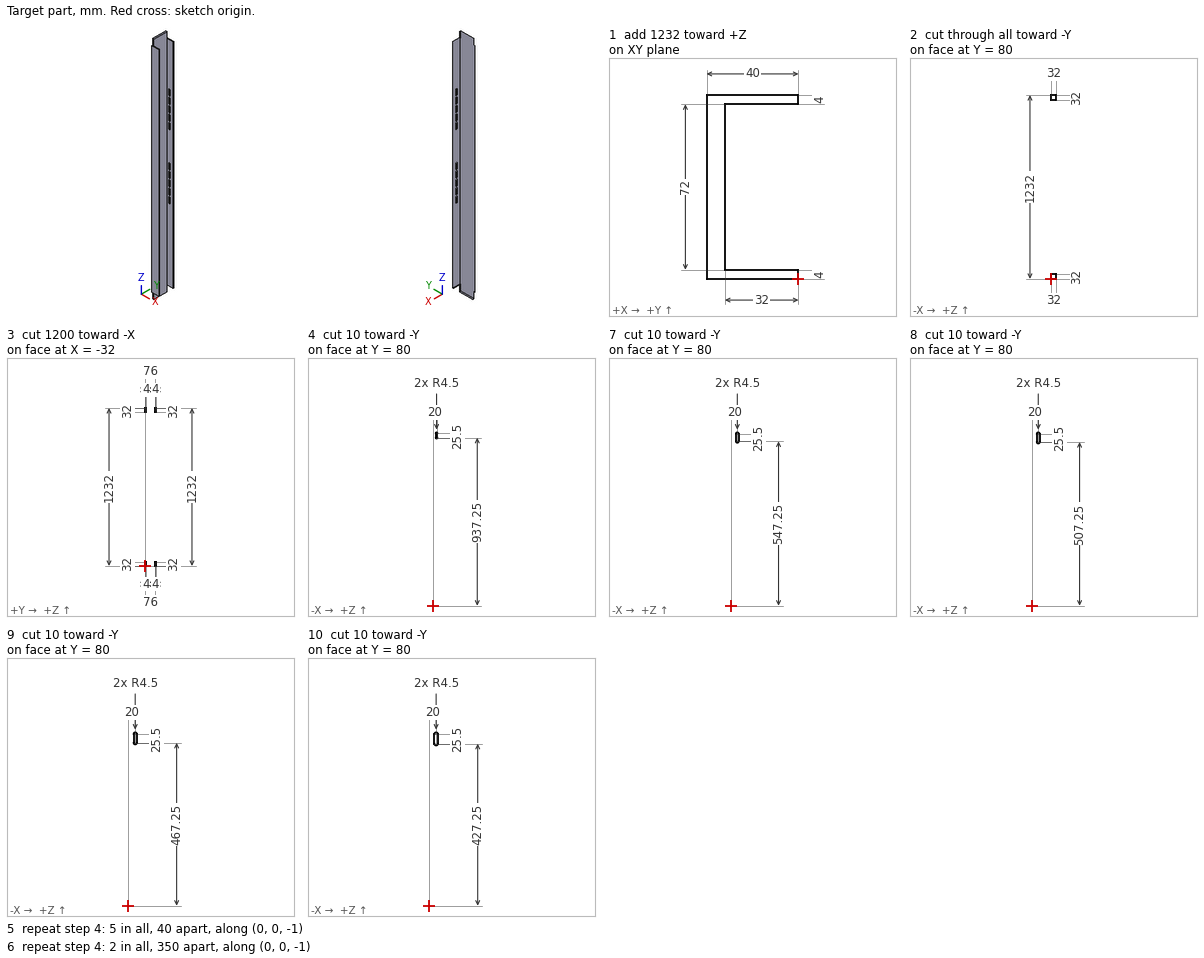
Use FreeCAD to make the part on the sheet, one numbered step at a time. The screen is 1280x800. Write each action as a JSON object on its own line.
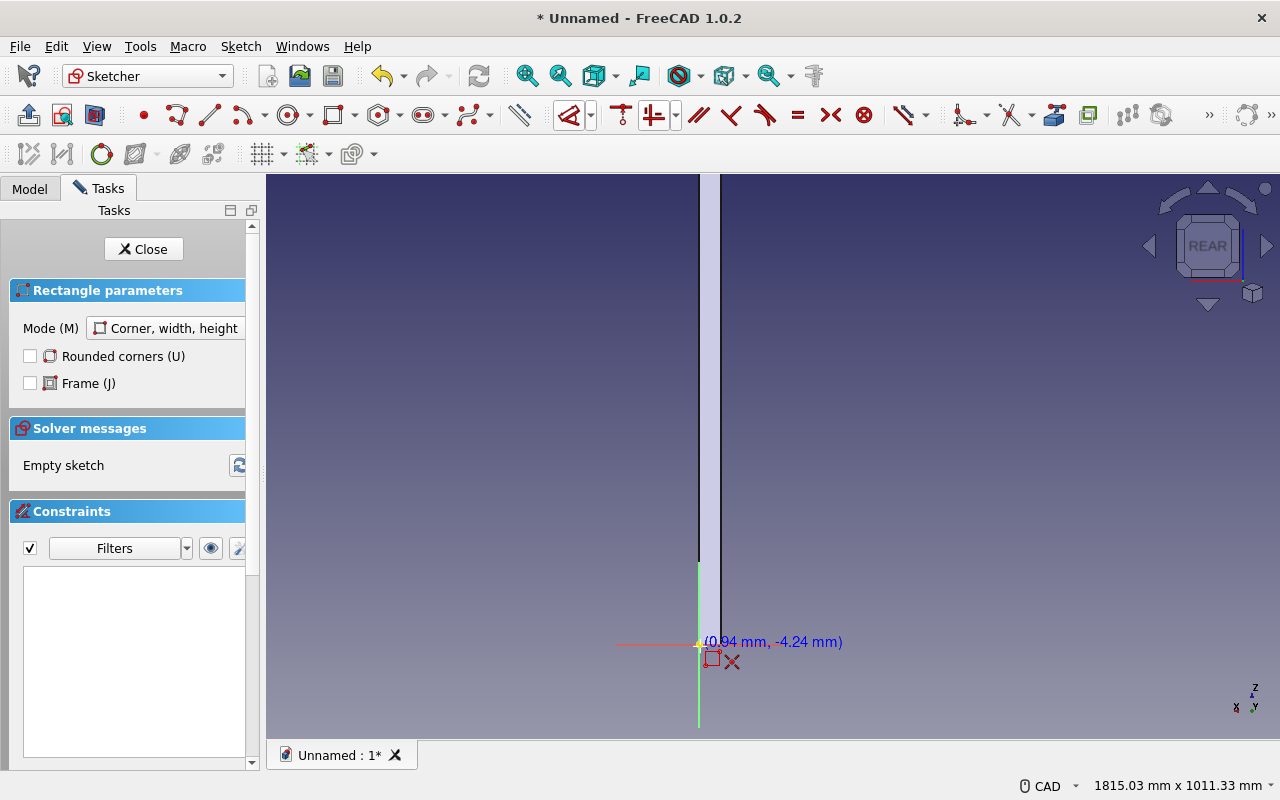
{"action": "left_click", "coordinate": [699, 645]}
{"action": "mouse_move", "coordinate": [717, 627]}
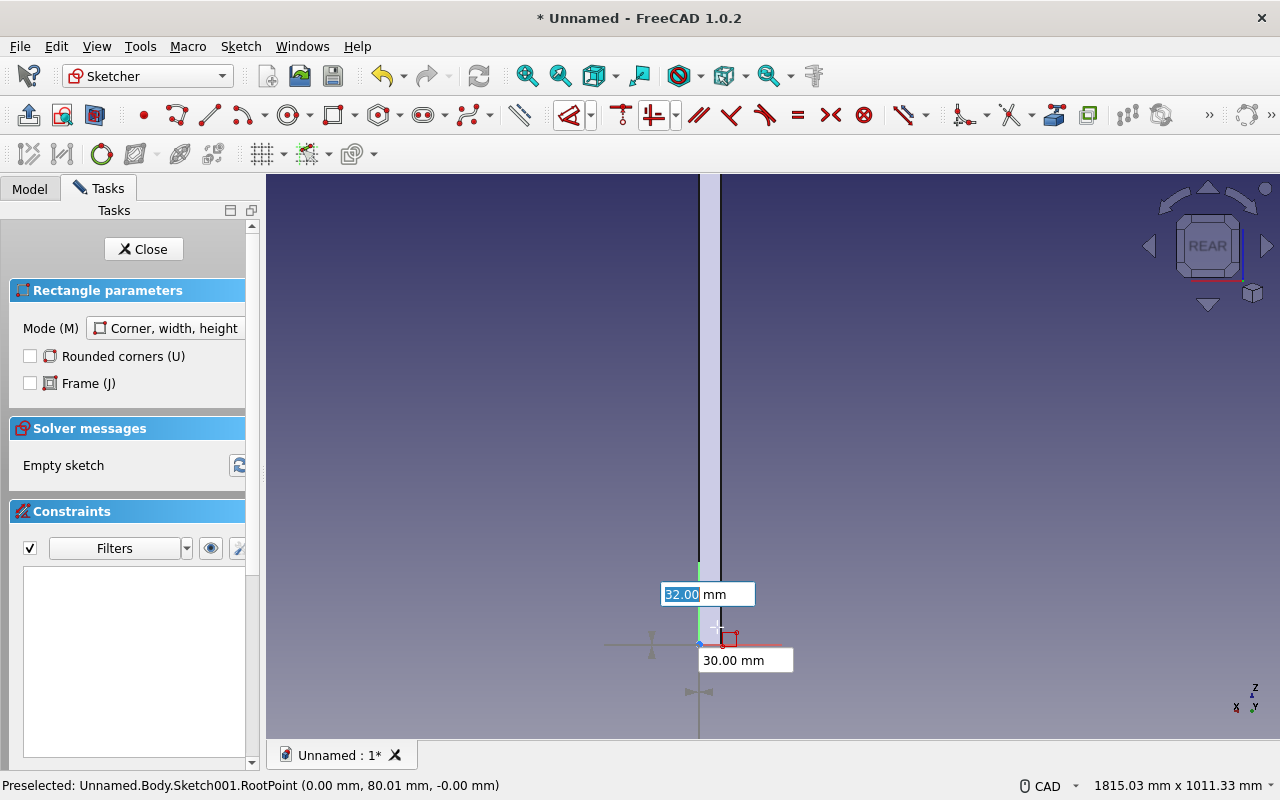
{"action": "type", "text": "32"}
{"action": "key", "text": "Tab"}
{"action": "type", "text": "32"}
{"action": "key", "text": "Return"}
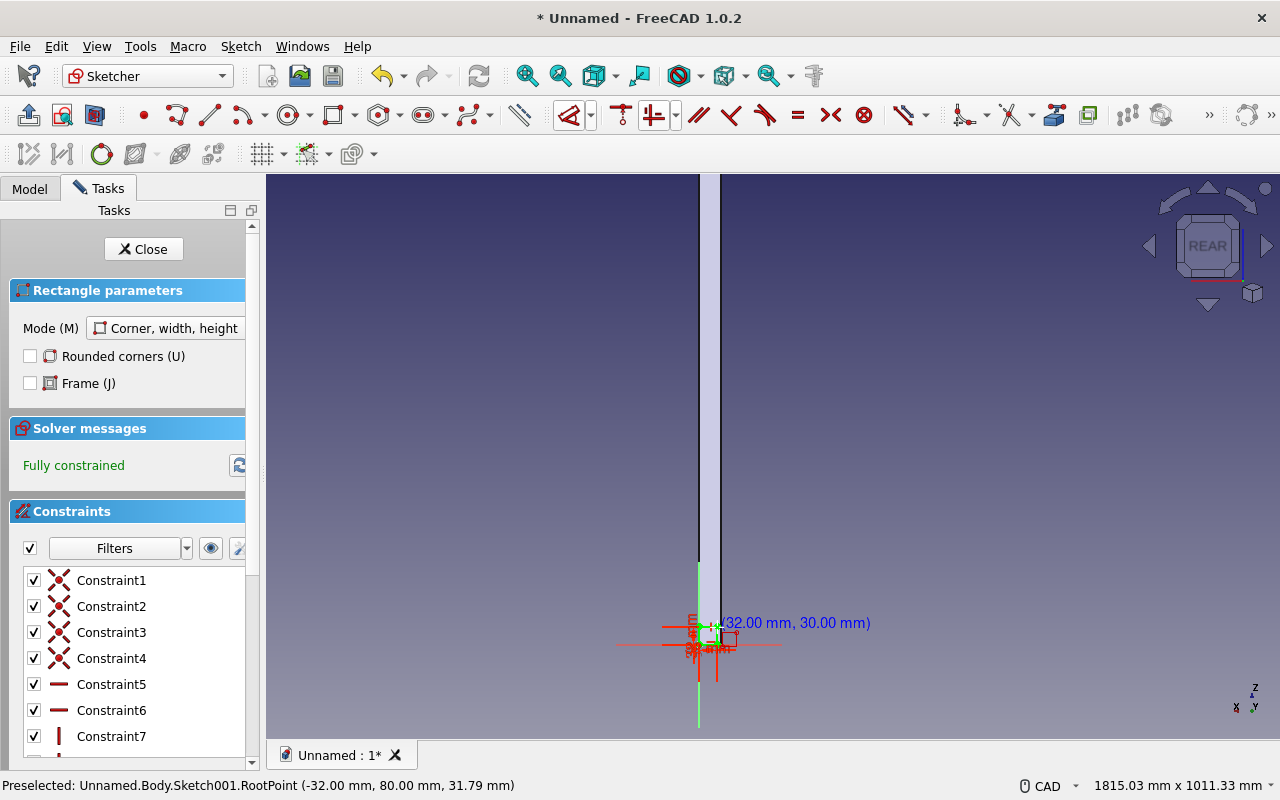
{"action": "scroll", "coordinate": [700, 646], "scroll_direction": "down", "scroll_amount": 3}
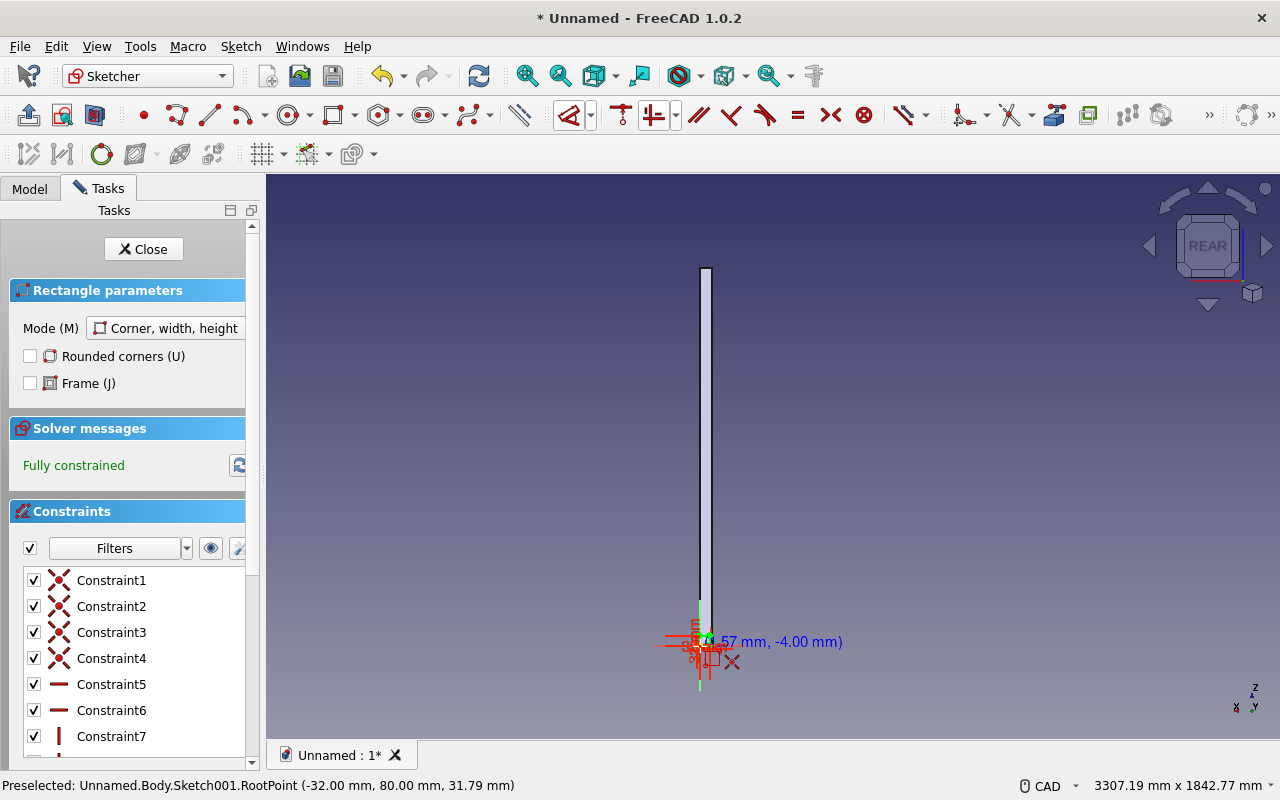
{"action": "scroll", "coordinate": [700, 268], "scroll_direction": "up", "scroll_amount": 3}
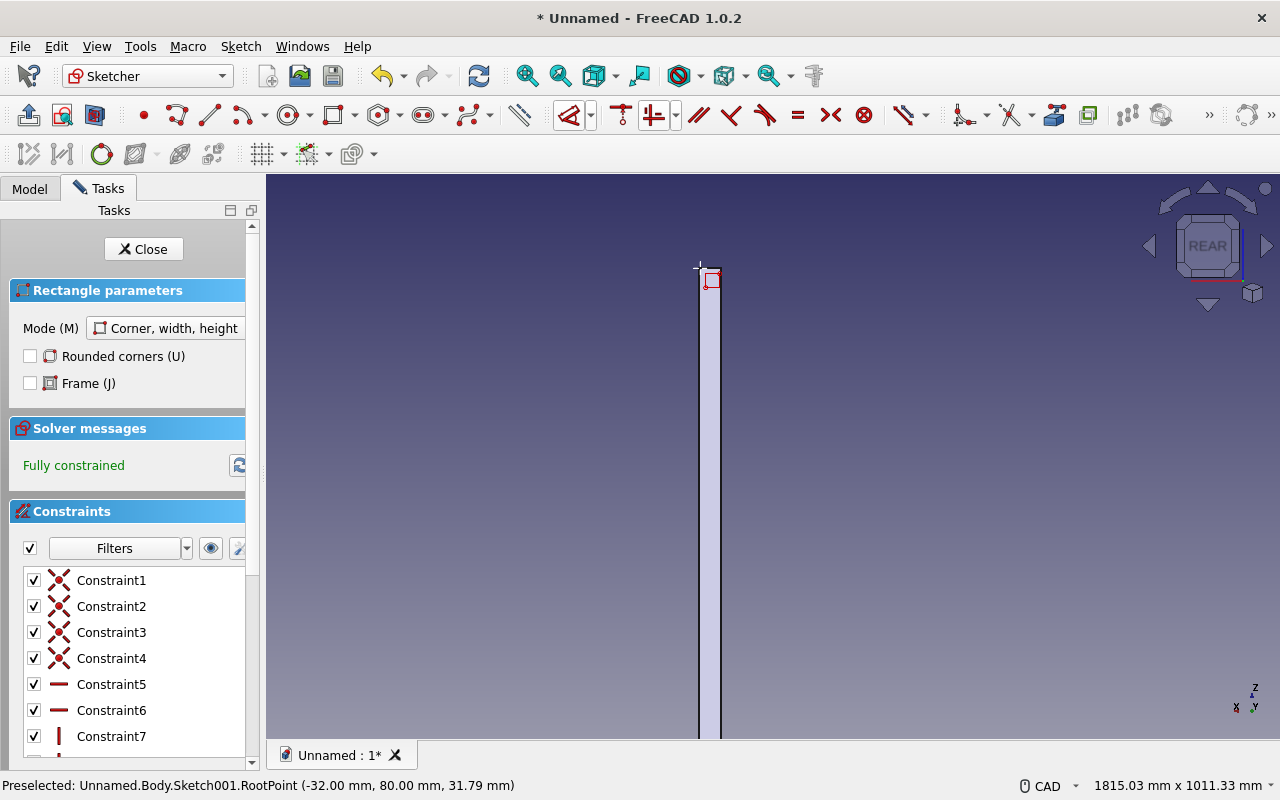
{"action": "left_click", "coordinate": [699, 268]}
{"action": "mouse_move", "coordinate": [717, 286]}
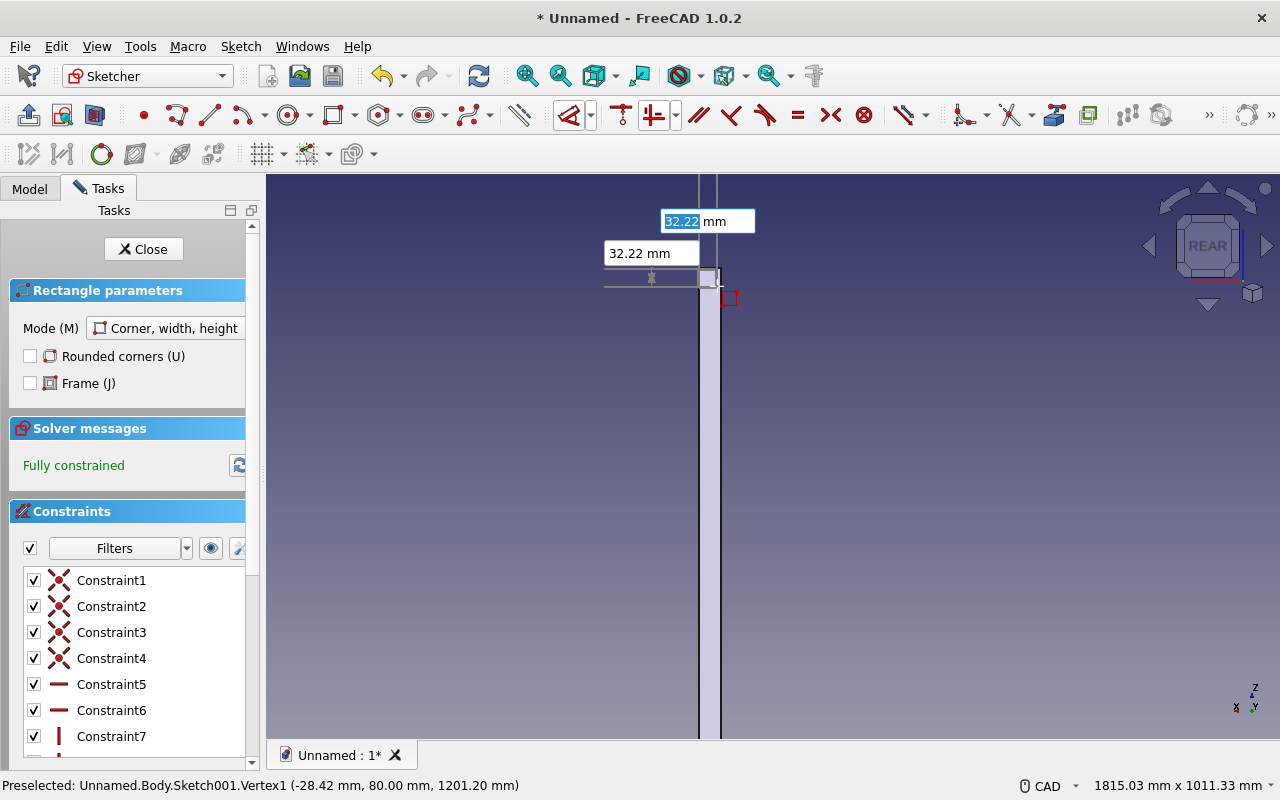
{"action": "type", "text": "32"}
{"action": "key", "text": "Tab"}
{"action": "type", "text": "32"}
{"action": "key", "text": "Return"}
{"action": "key", "text": "Escape"}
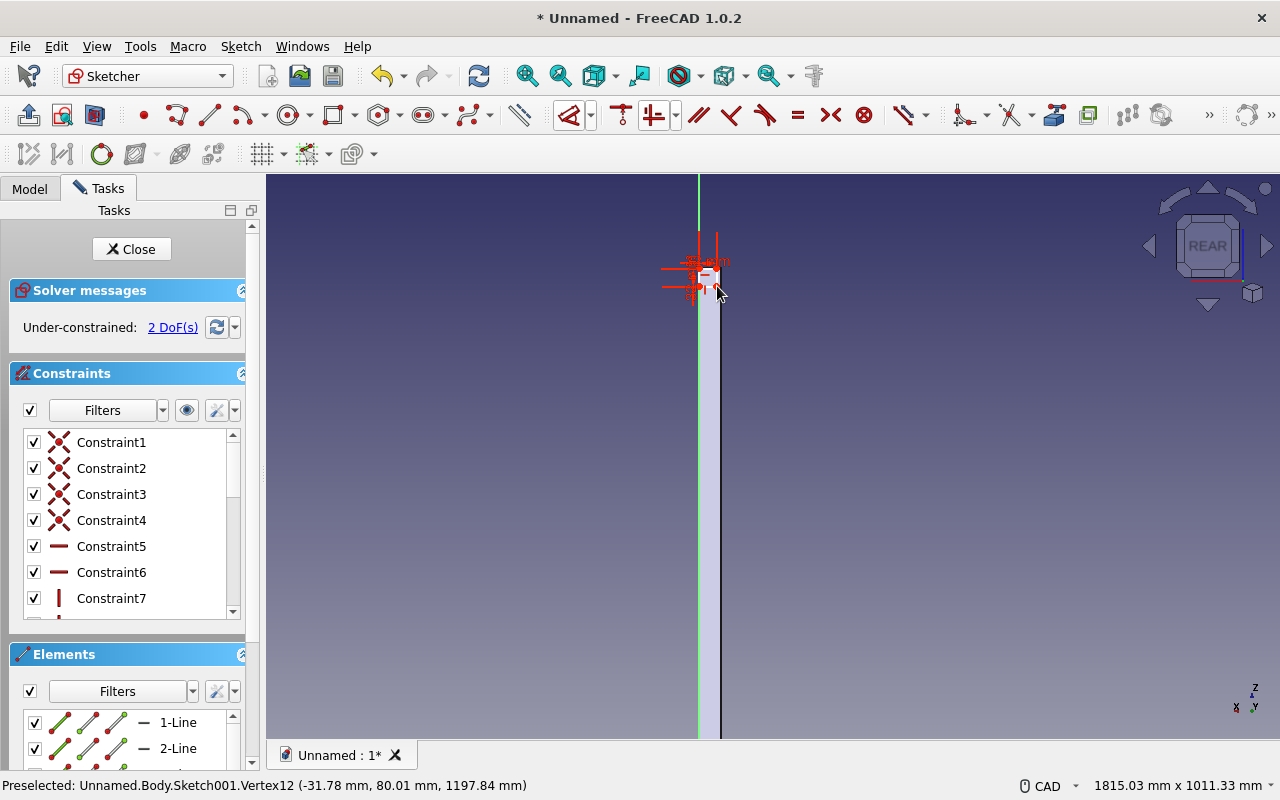
{"action": "left_click", "coordinate": [699, 269]}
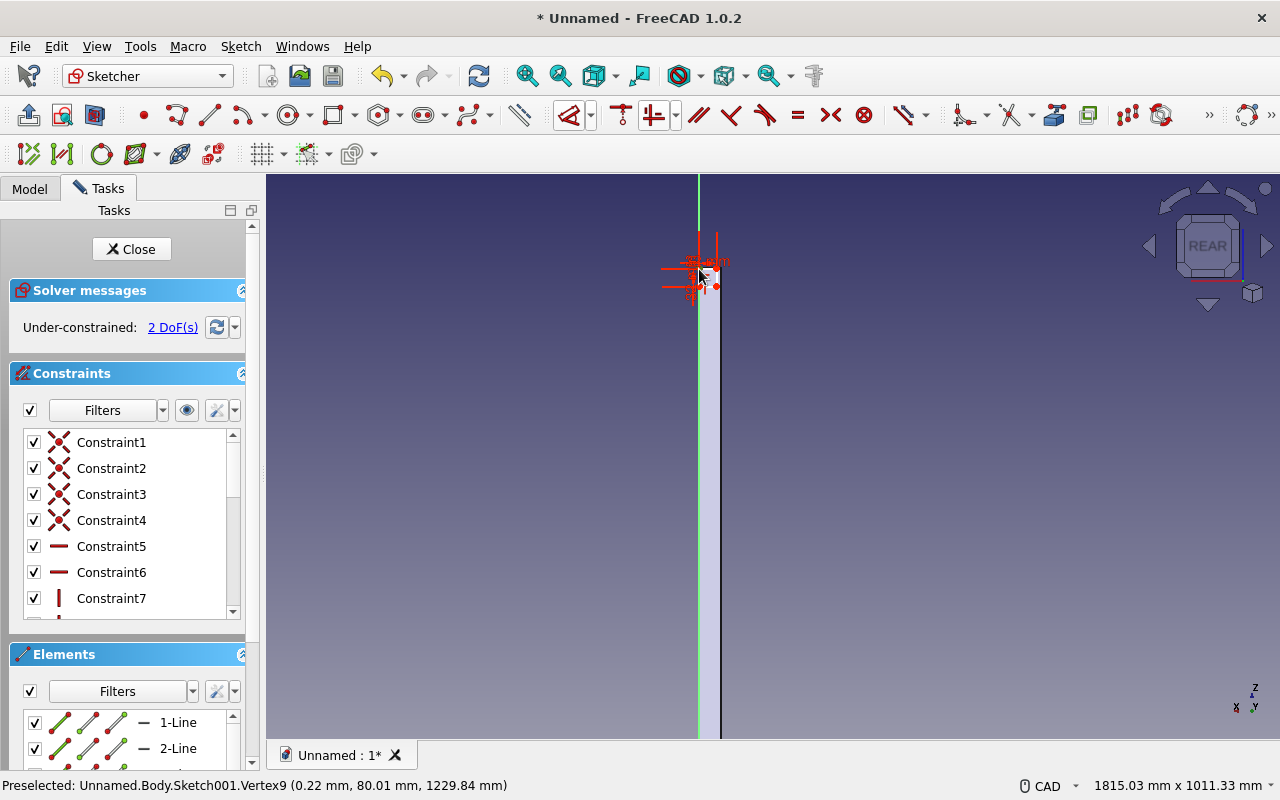
{"action": "left_click", "coordinate": [699, 675]}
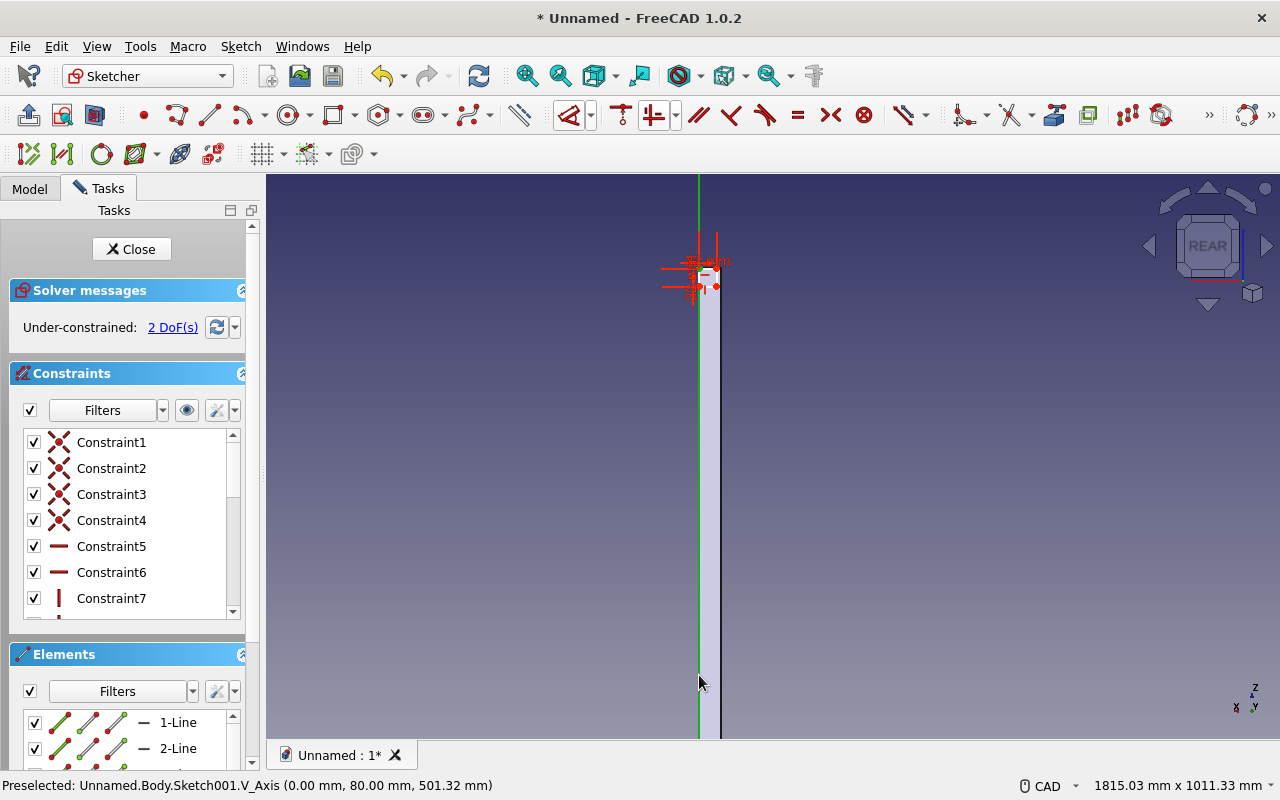
{"action": "left_click", "coordinate": [621, 116]}